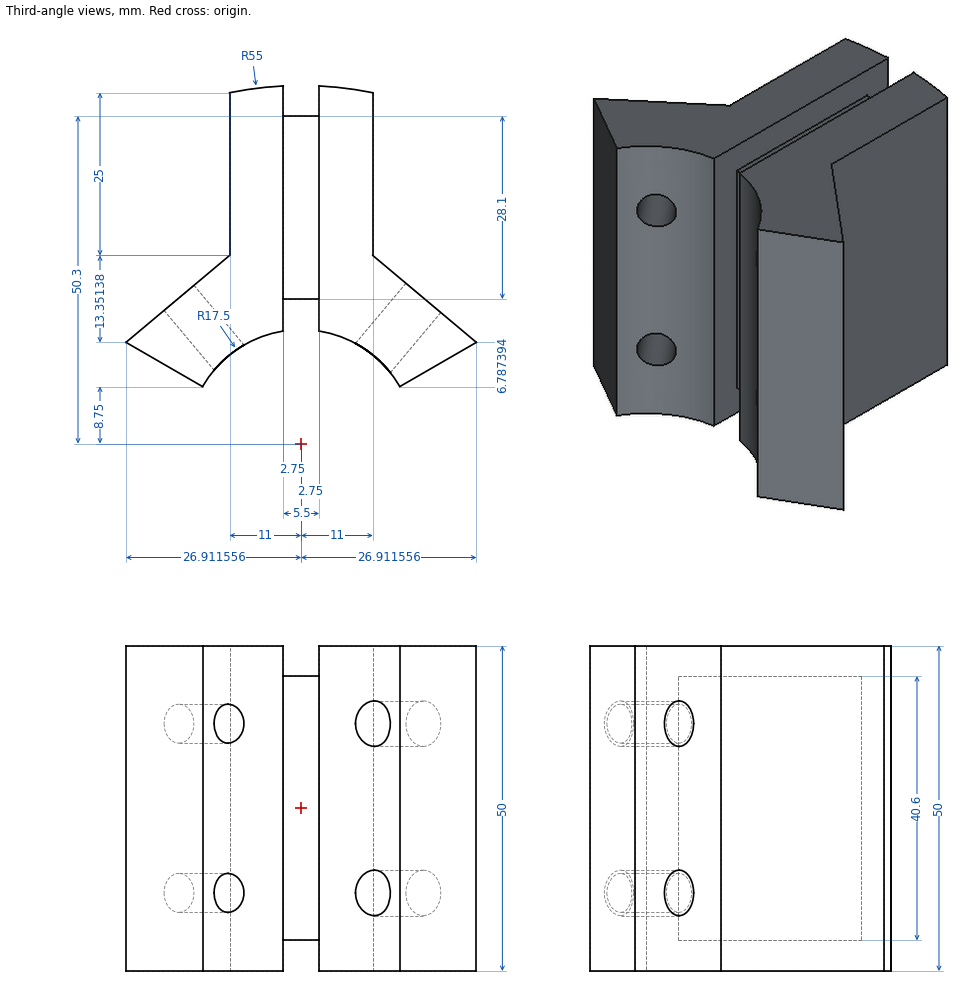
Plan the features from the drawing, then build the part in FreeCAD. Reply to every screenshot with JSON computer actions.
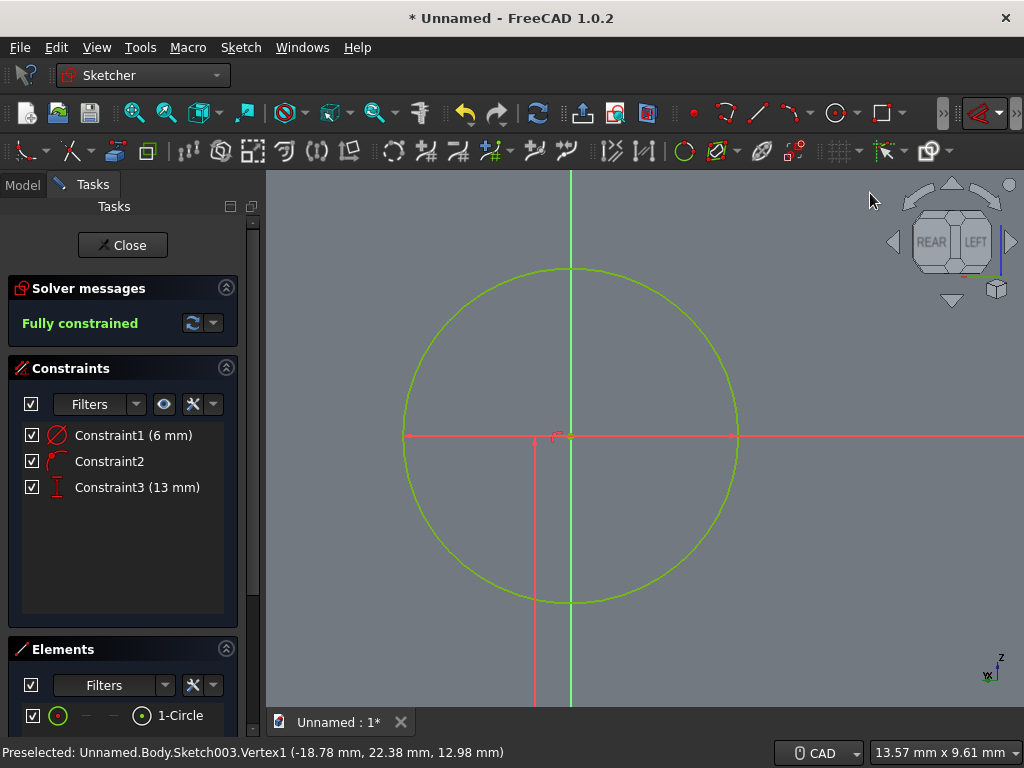
{"action": "left_click", "coordinate": [123, 245]}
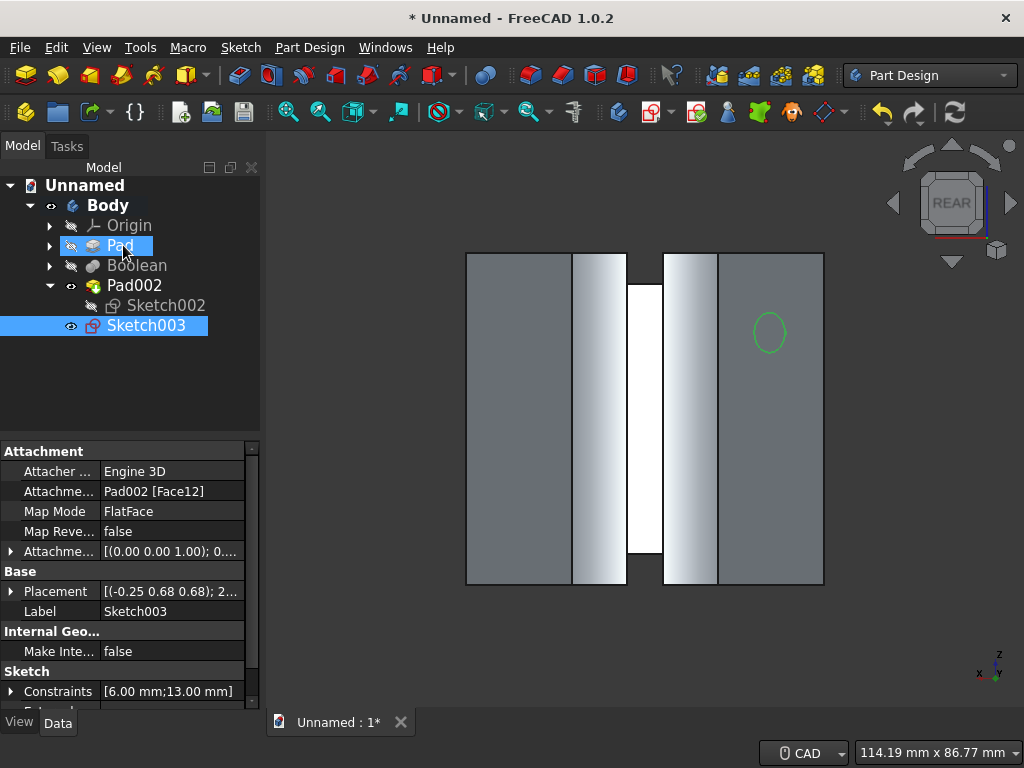
{"action": "left_click", "coordinate": [240, 76]}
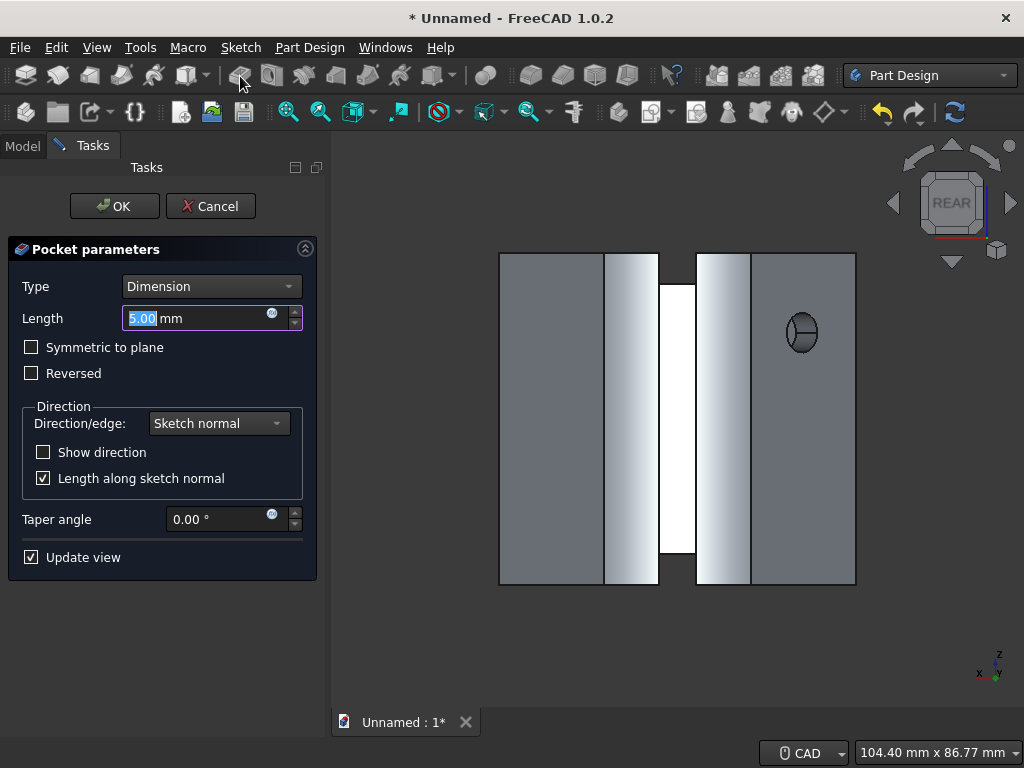
{"action": "left_click", "coordinate": [212, 286]}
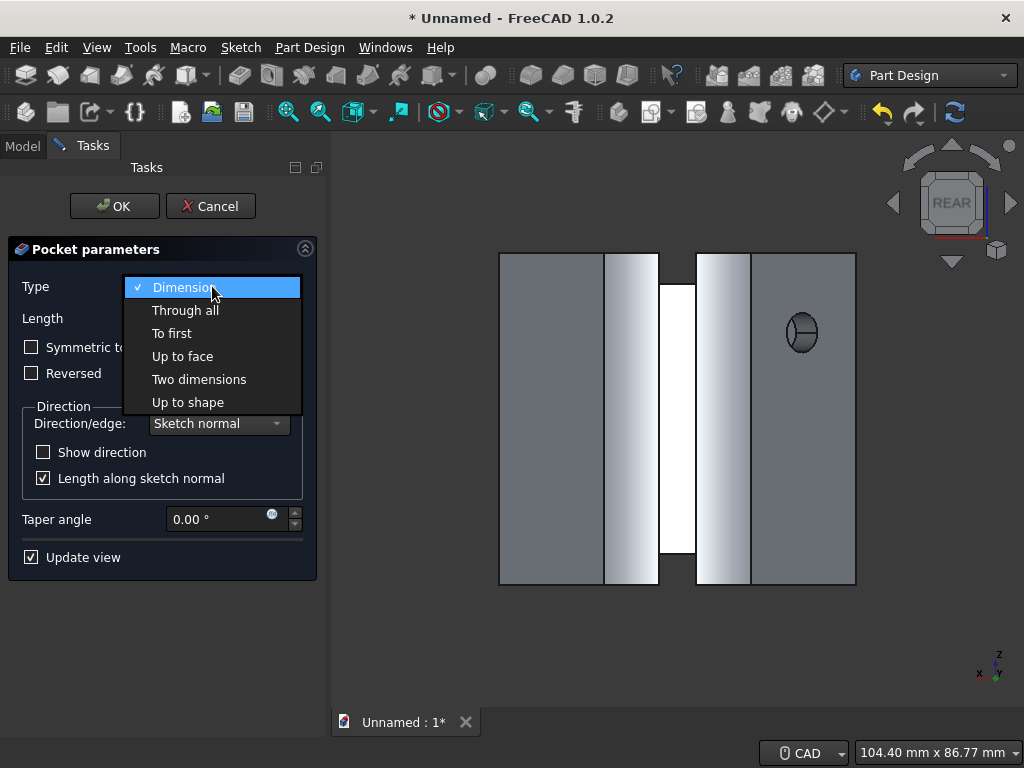
{"action": "left_click", "coordinate": [212, 310]}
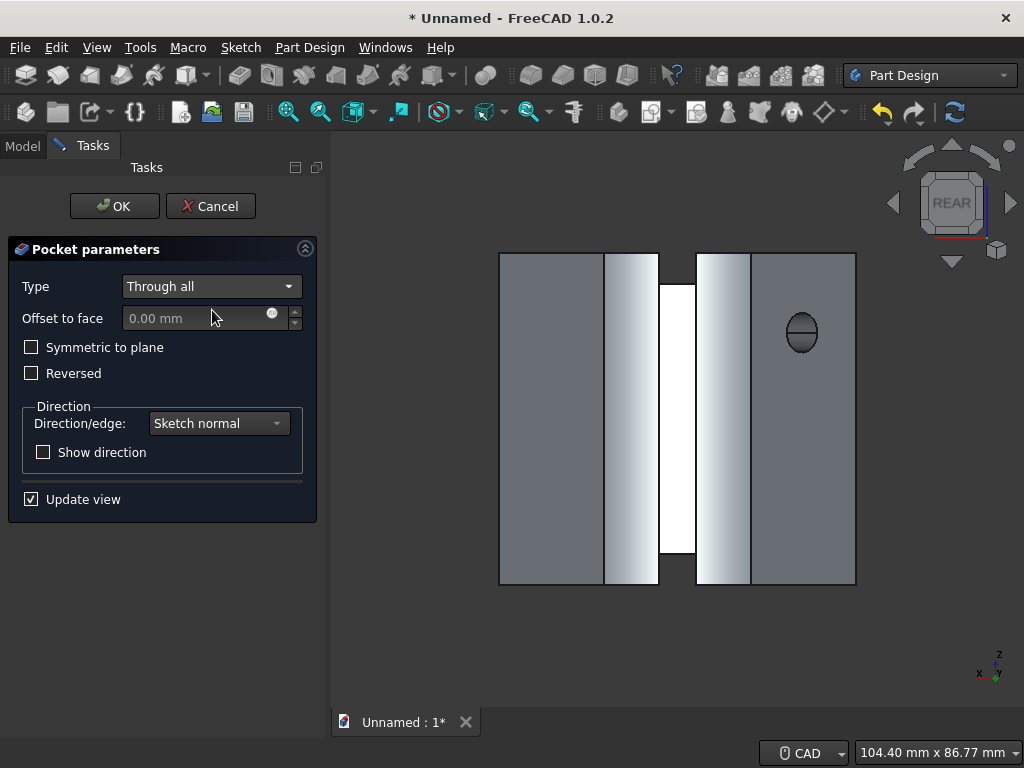
{"action": "left_click", "coordinate": [115, 206]}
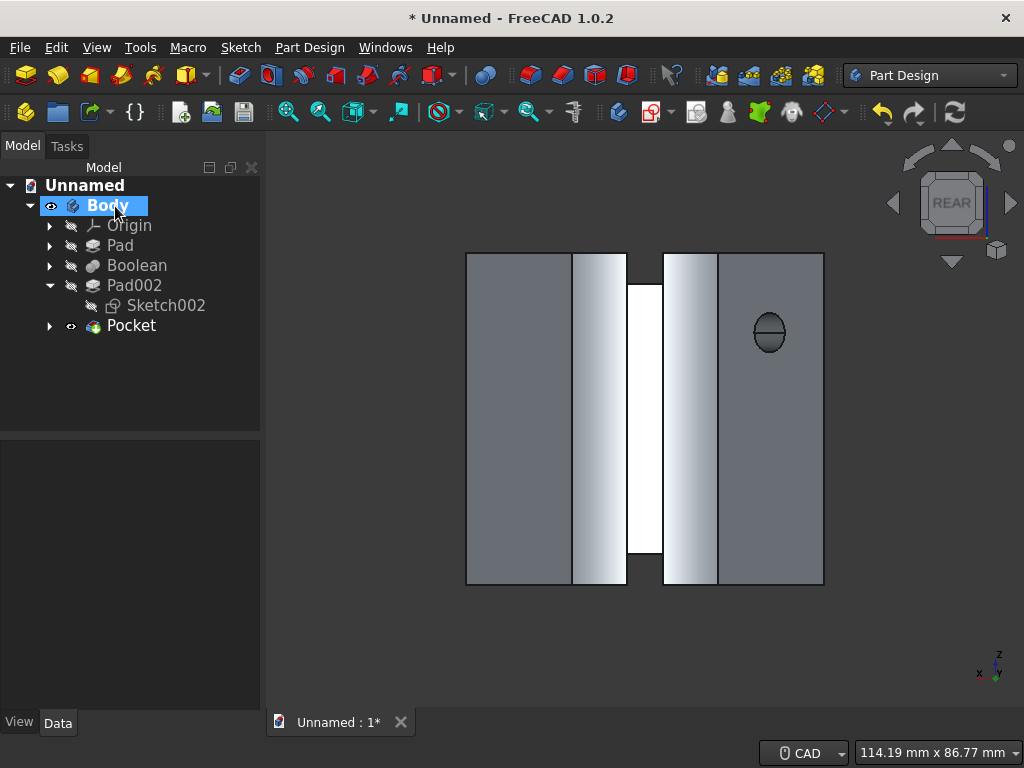
{"action": "left_click", "coordinate": [771, 465]}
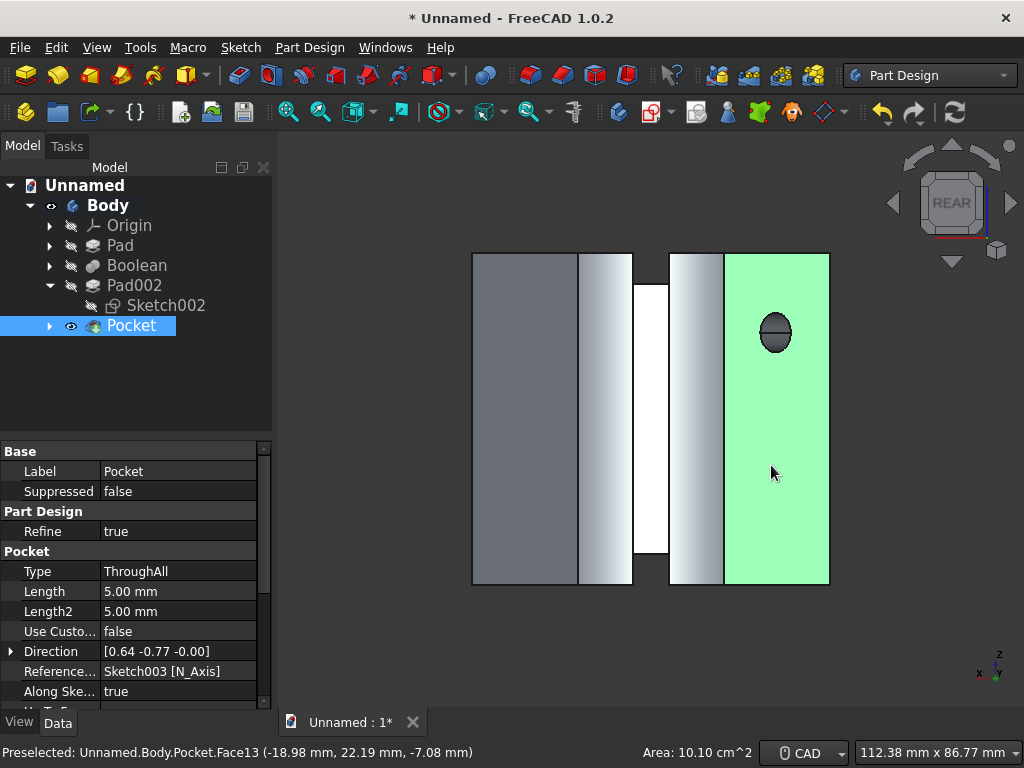
{"action": "left_click", "coordinate": [652, 112]}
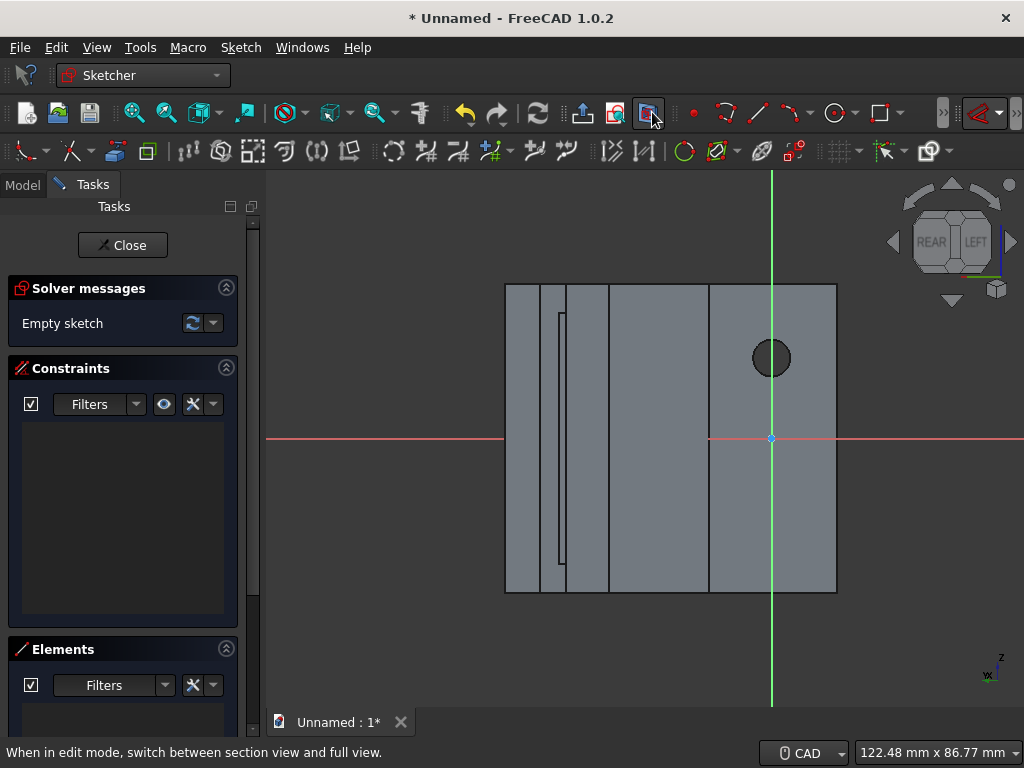
{"action": "scroll", "coordinate": [796, 529], "scroll_direction": "up", "scroll_amount": 11}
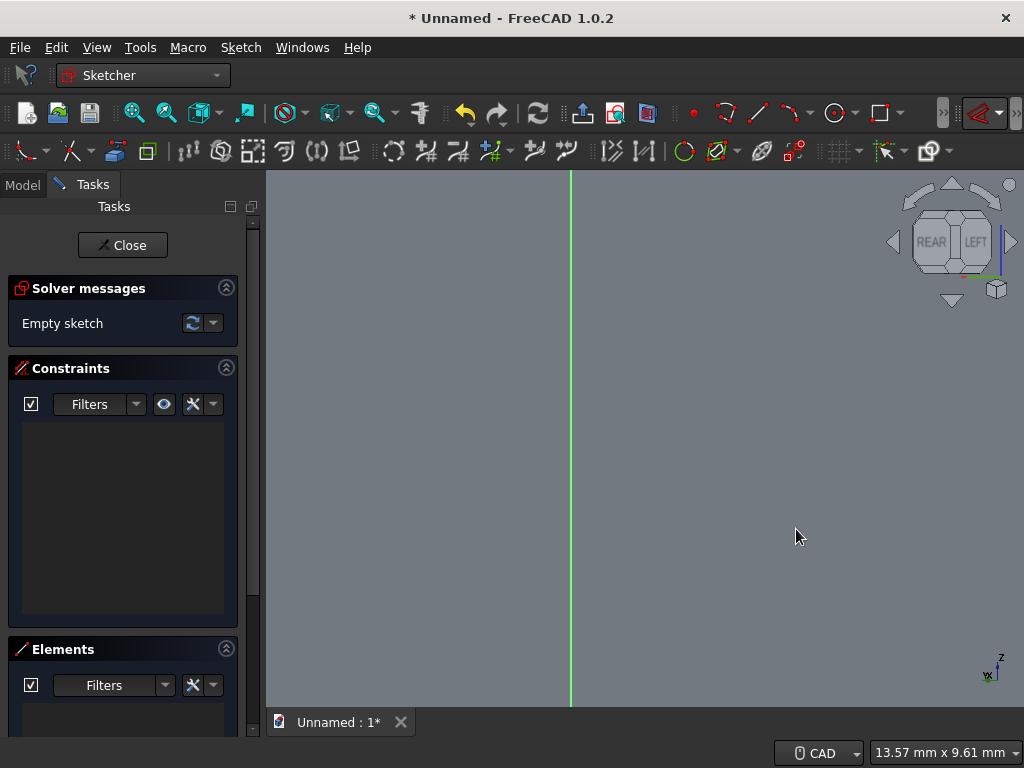
{"action": "left_click", "coordinate": [836, 114]}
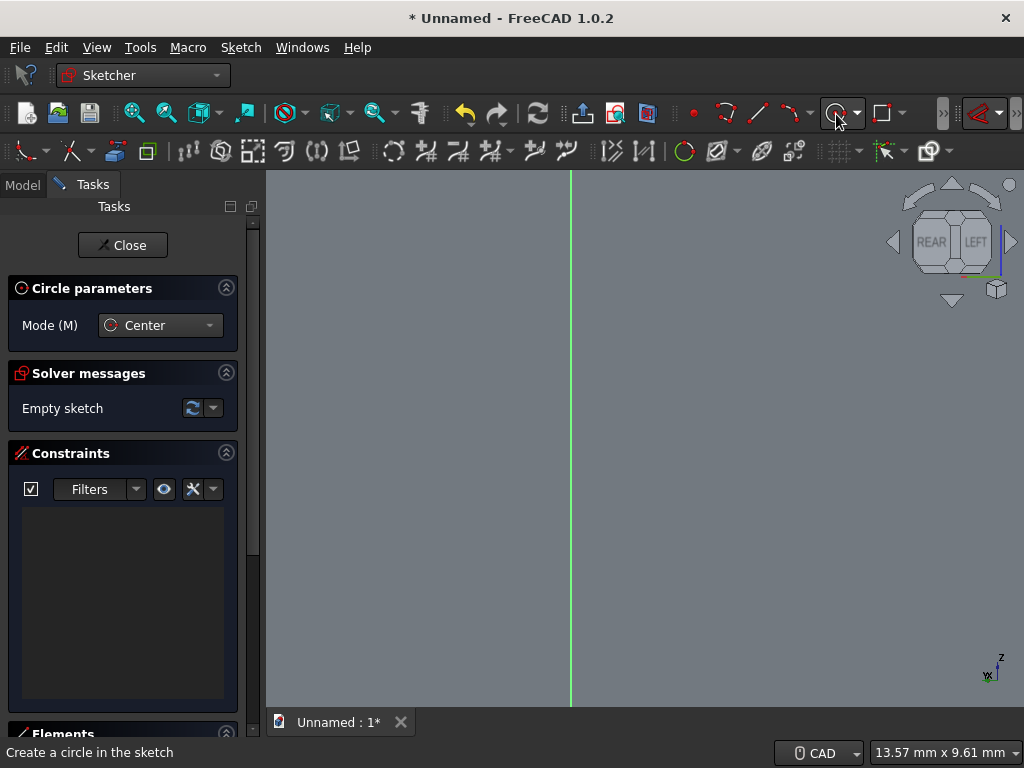
{"action": "left_click", "coordinate": [571, 433]}
{"action": "mouse_move", "coordinate": [689, 314]}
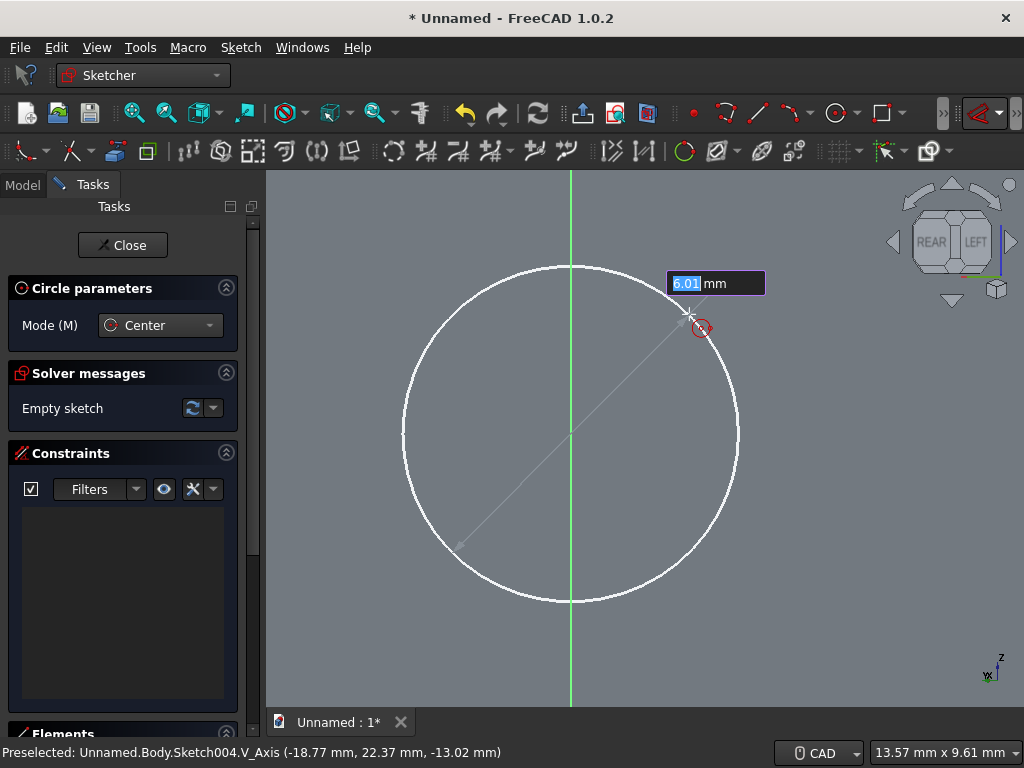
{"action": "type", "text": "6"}
{"action": "key", "text": "Return"}
{"action": "key", "text": "Escape"}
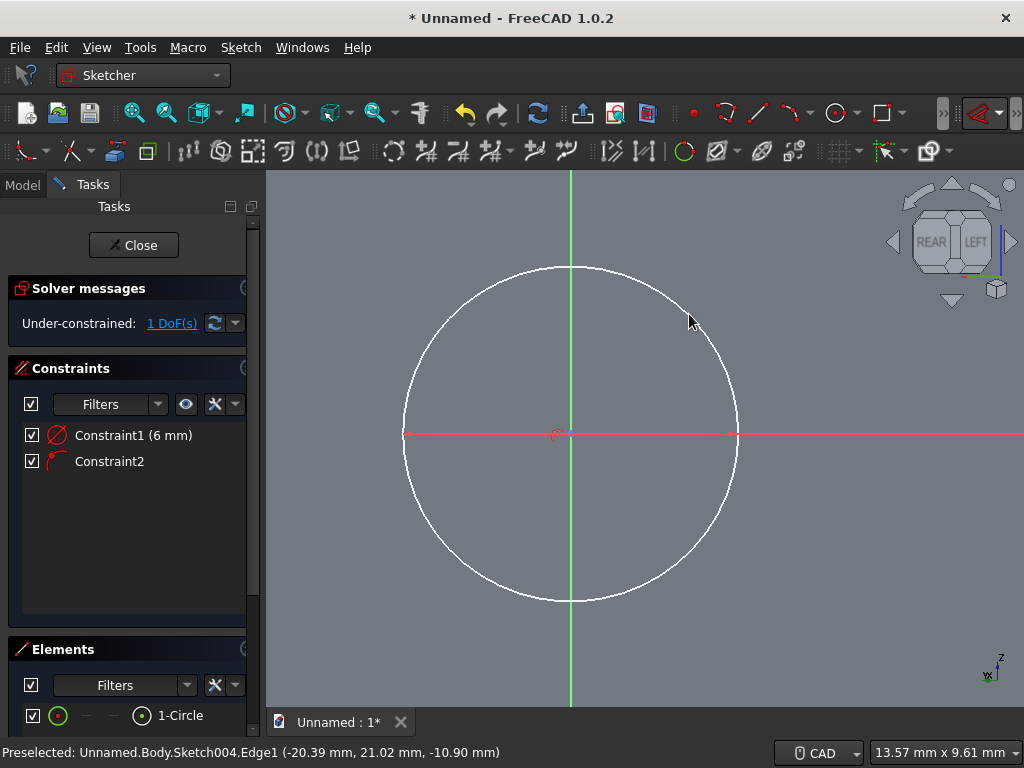
{"action": "left_click", "coordinate": [571, 434]}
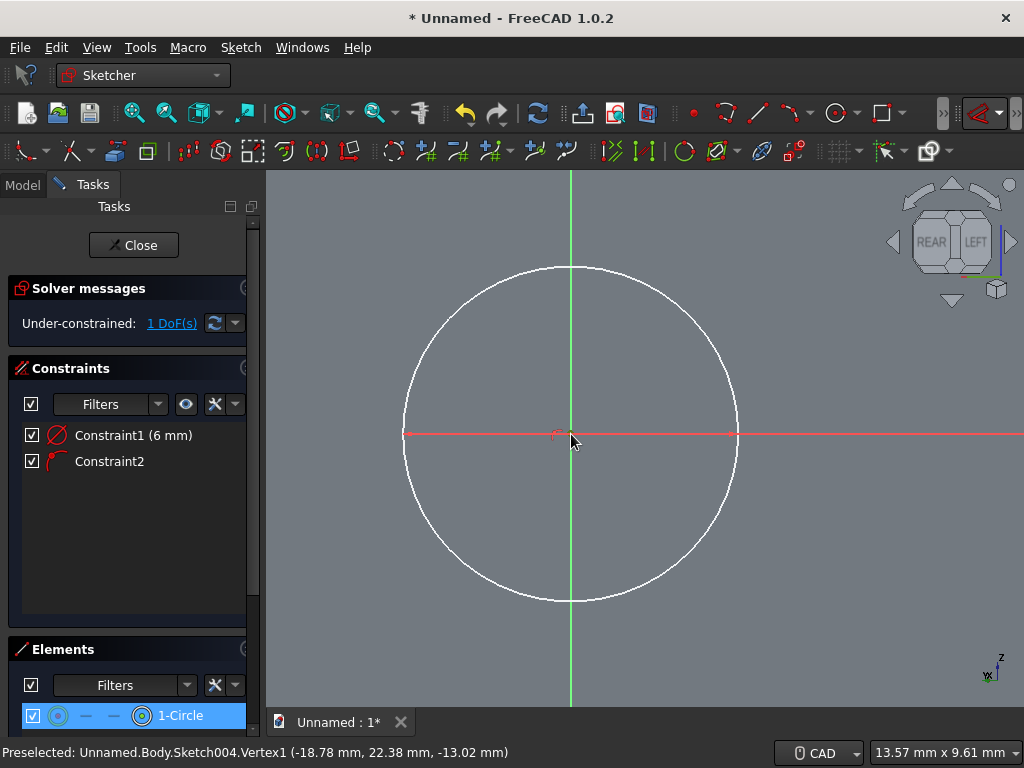
{"action": "left_click", "coordinate": [1002, 114]}